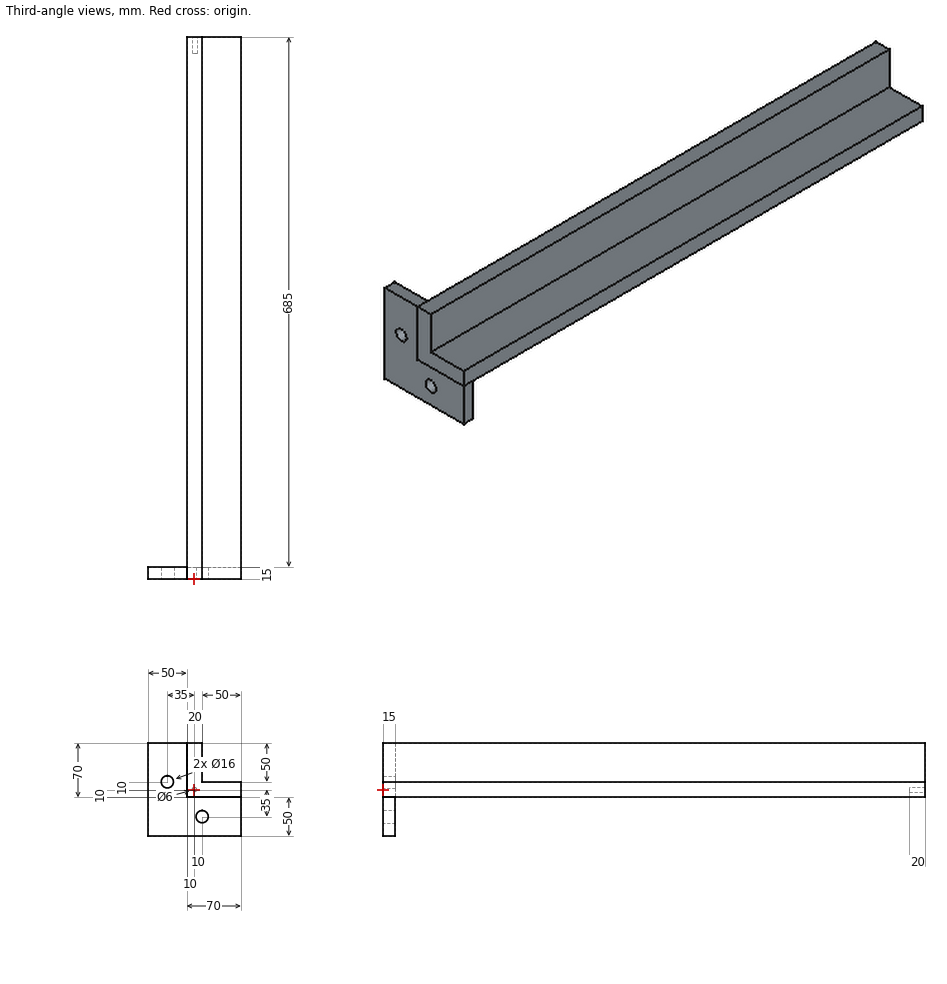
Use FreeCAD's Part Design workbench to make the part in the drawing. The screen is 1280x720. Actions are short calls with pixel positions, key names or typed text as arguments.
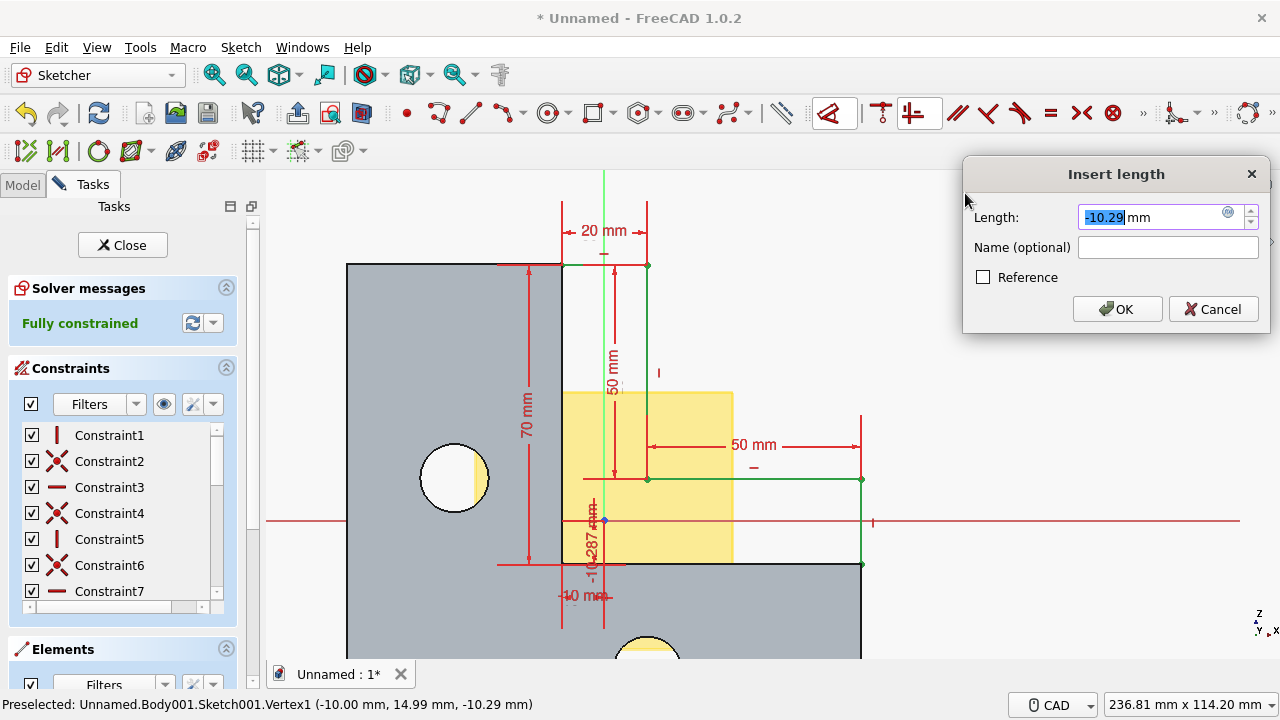
text(-10)
key(Return)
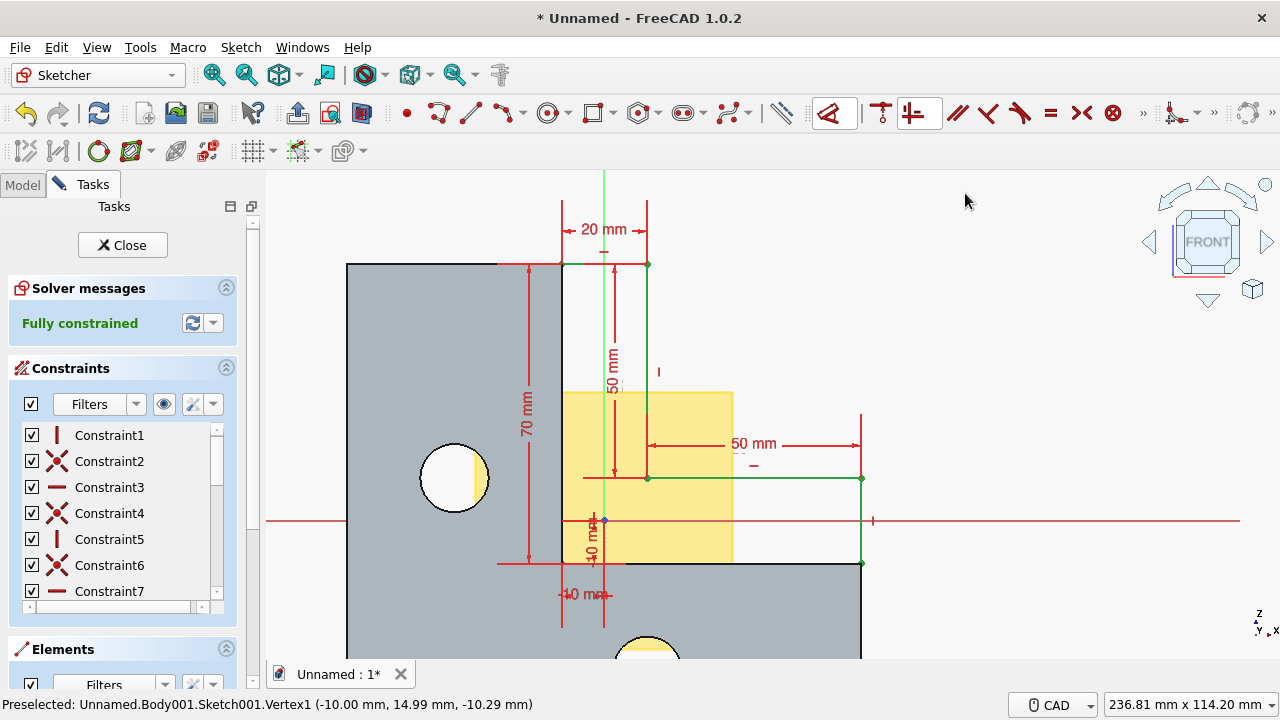
click(123, 245)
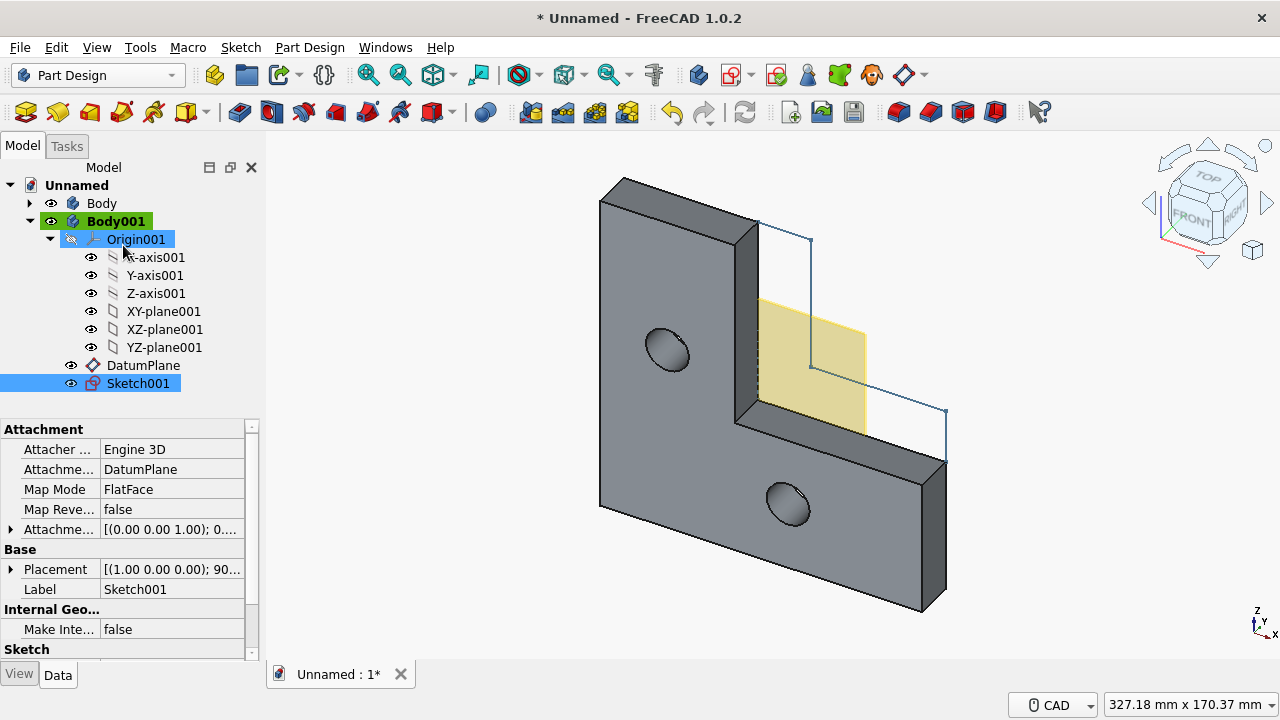
click(26, 112)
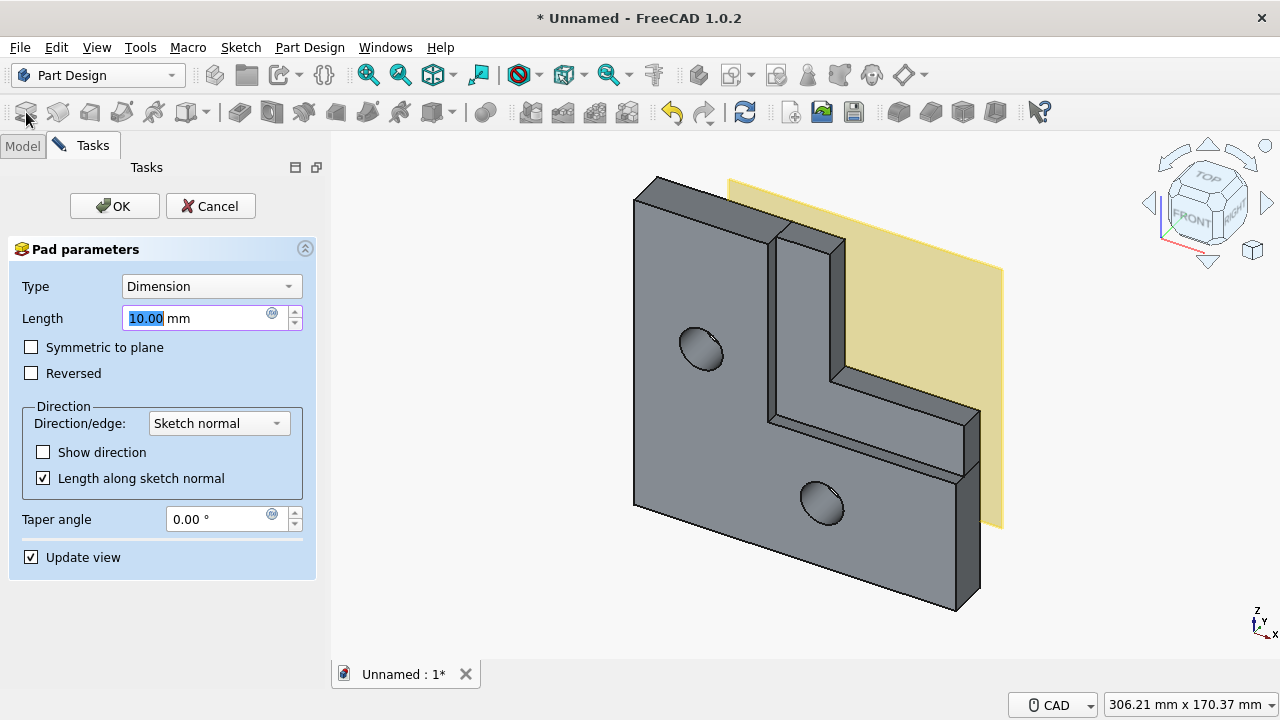
click(212, 286)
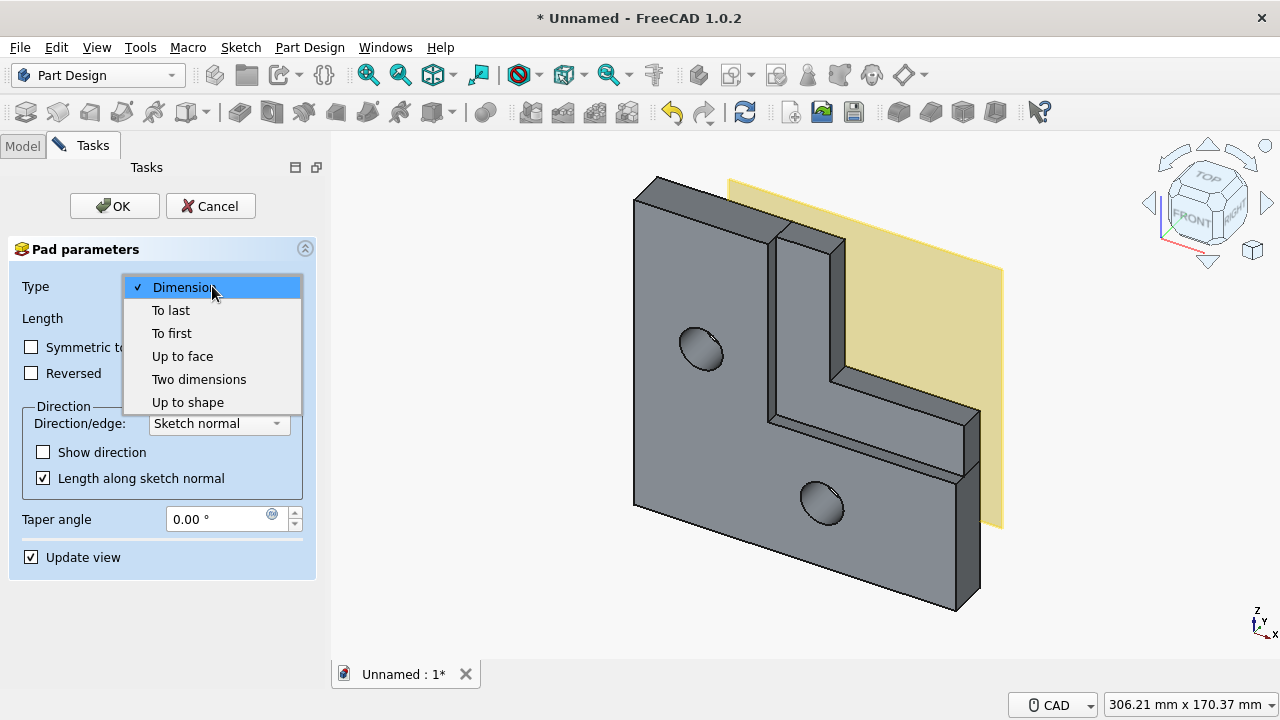
click(212, 380)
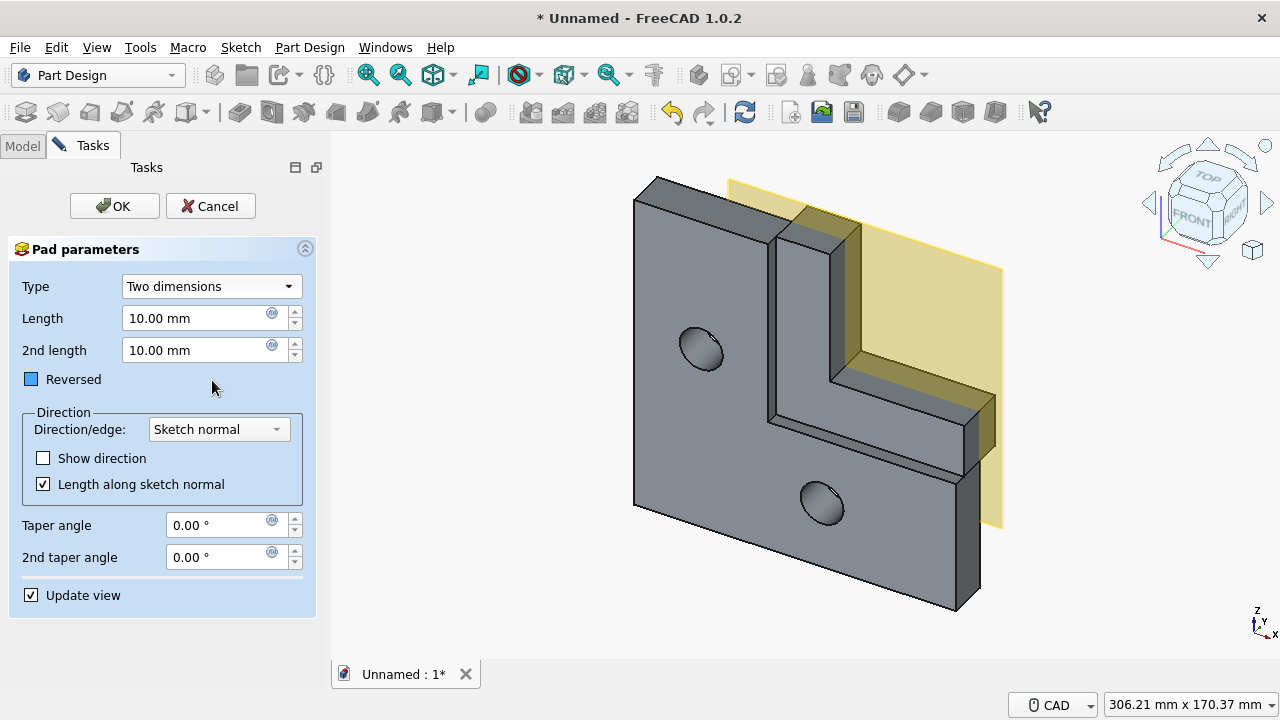
triple_click(204, 318)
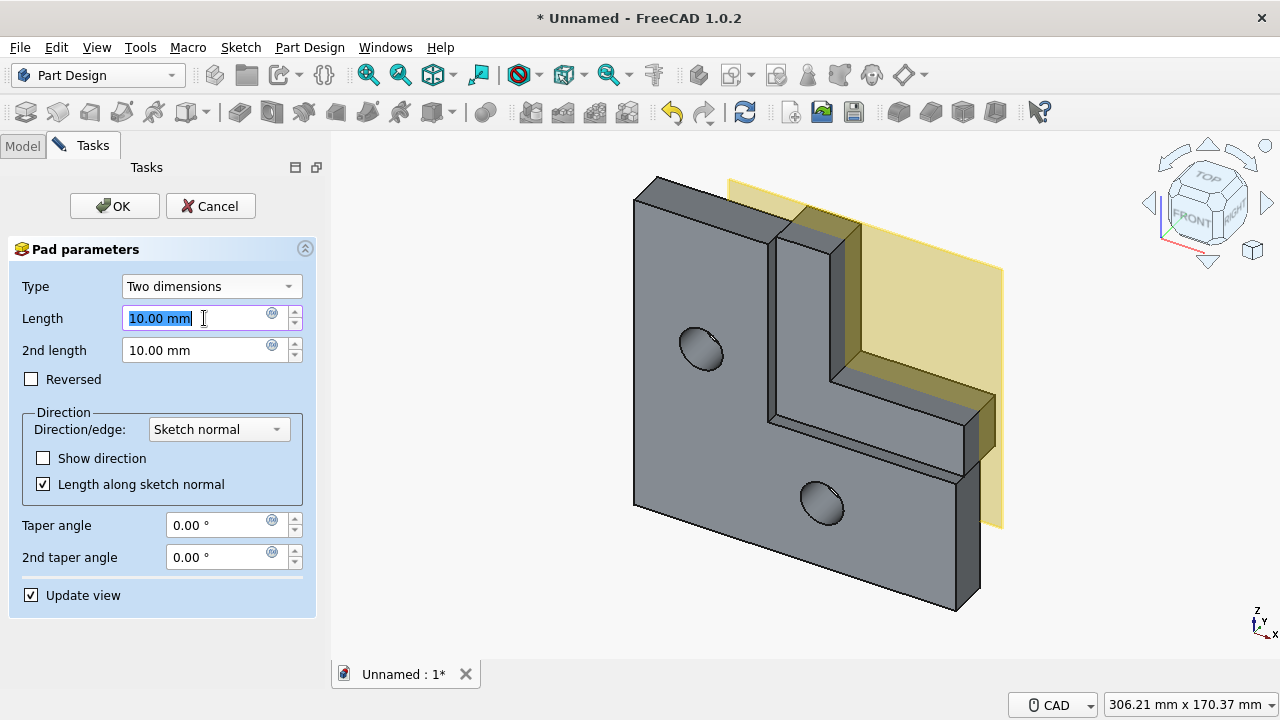
text(685)
key(Tab)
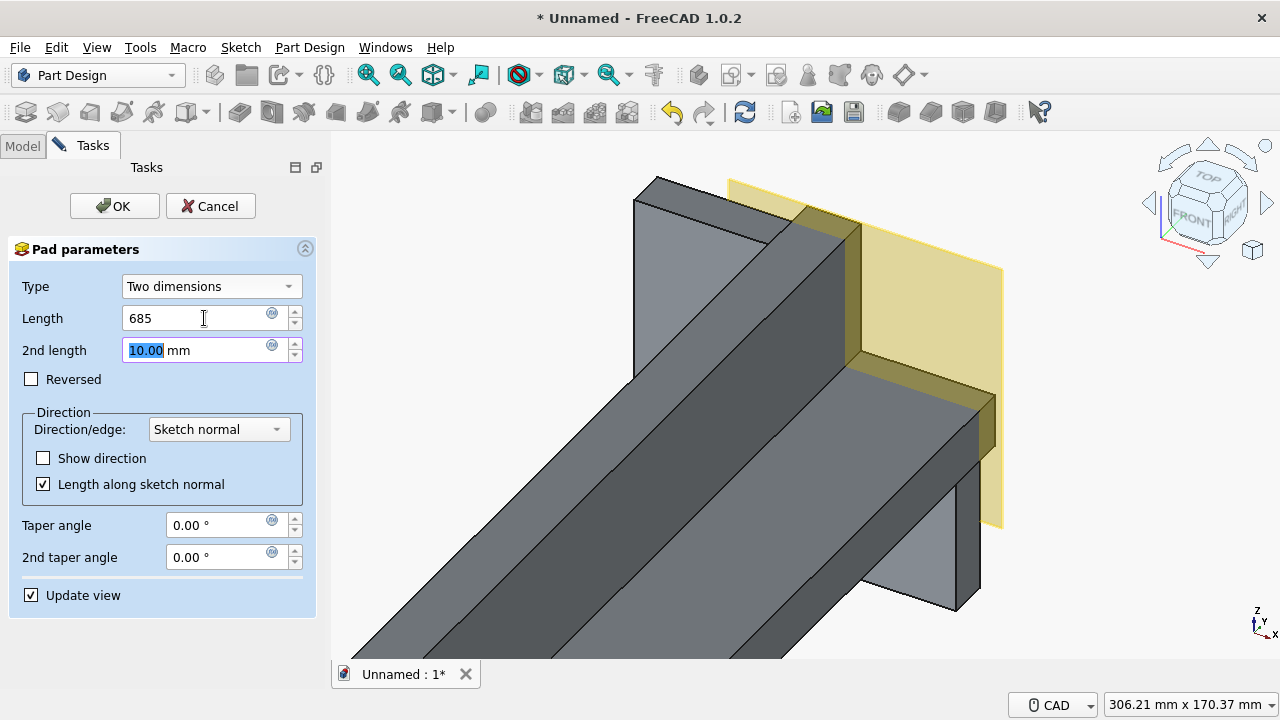
text(15)
key(Tab)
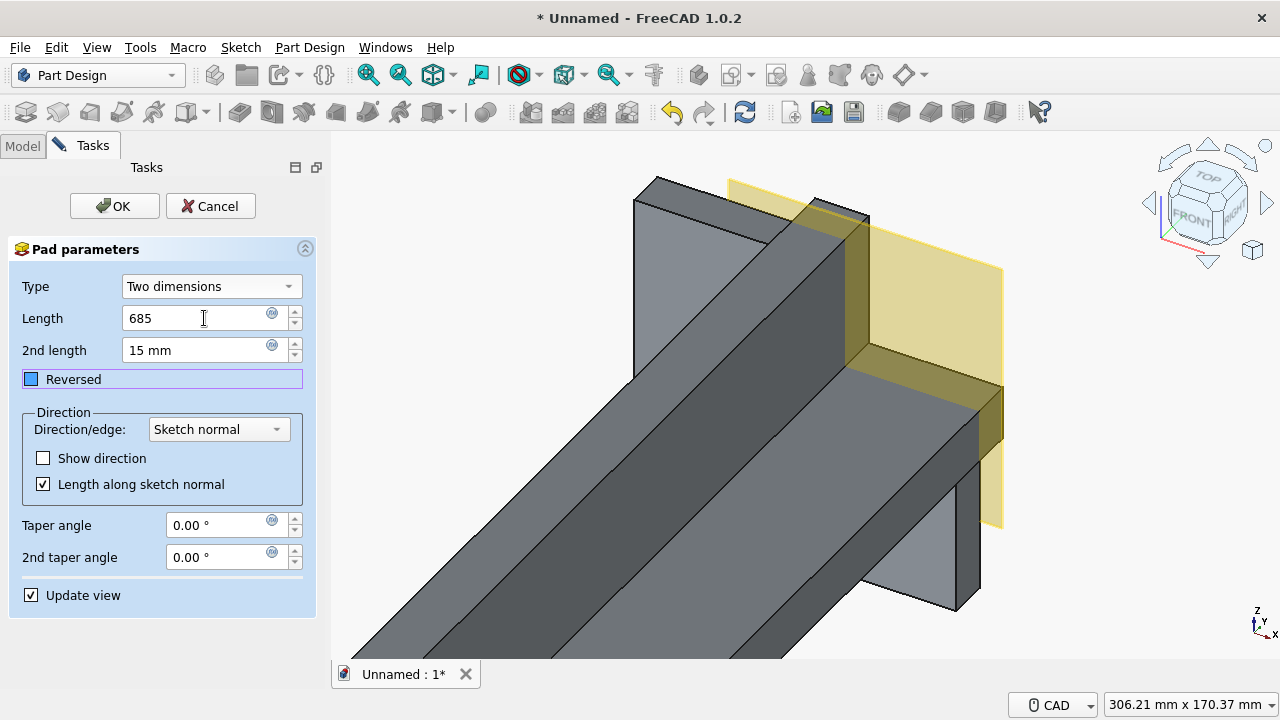
click(30, 379)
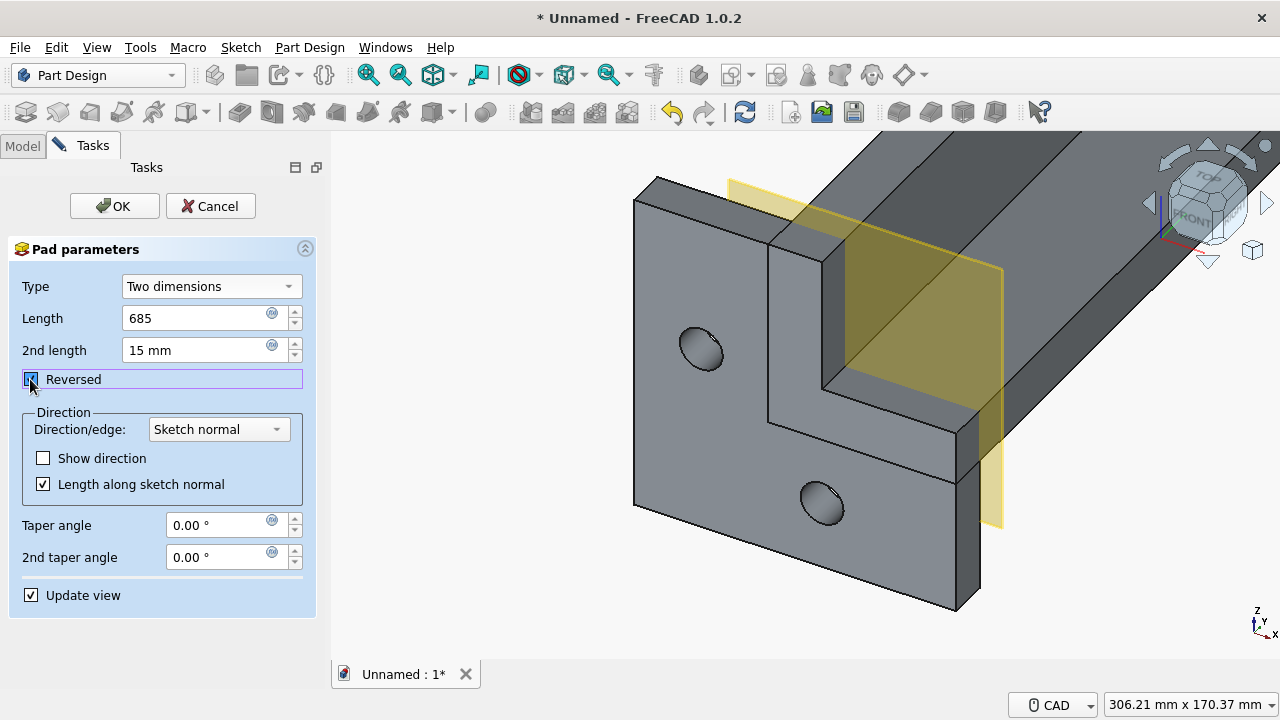
click(115, 206)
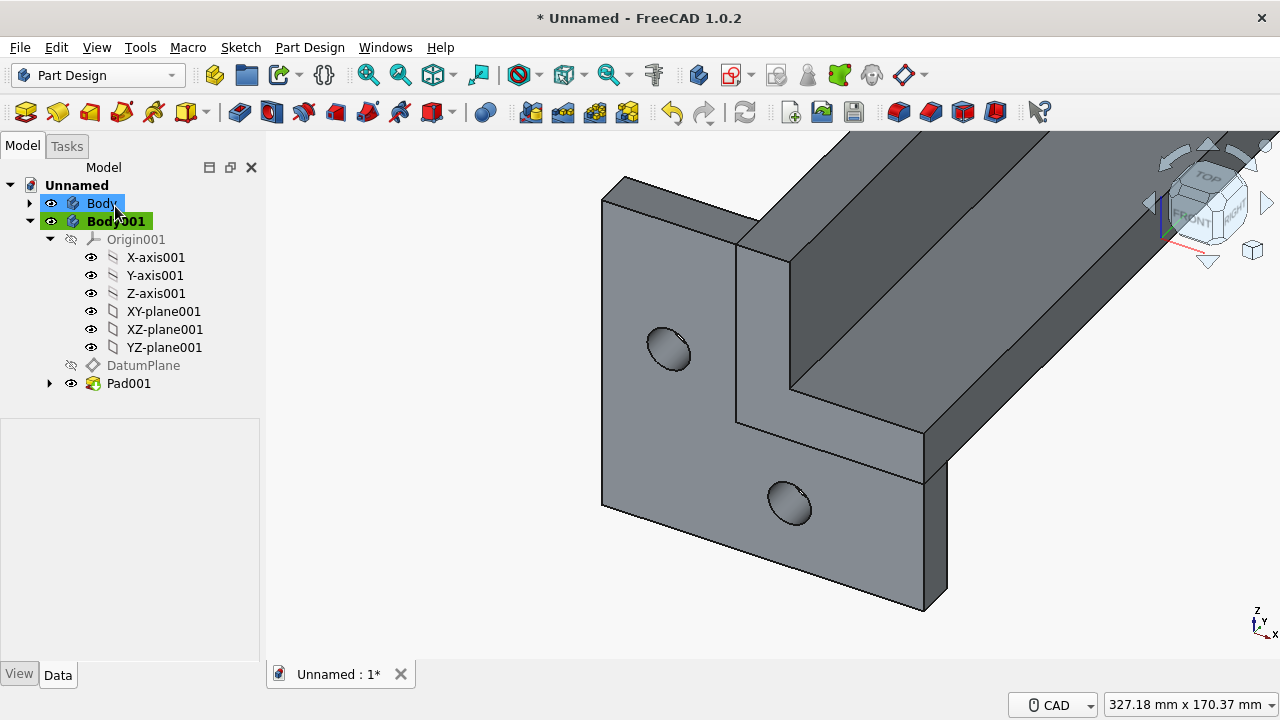
click(370, 76)